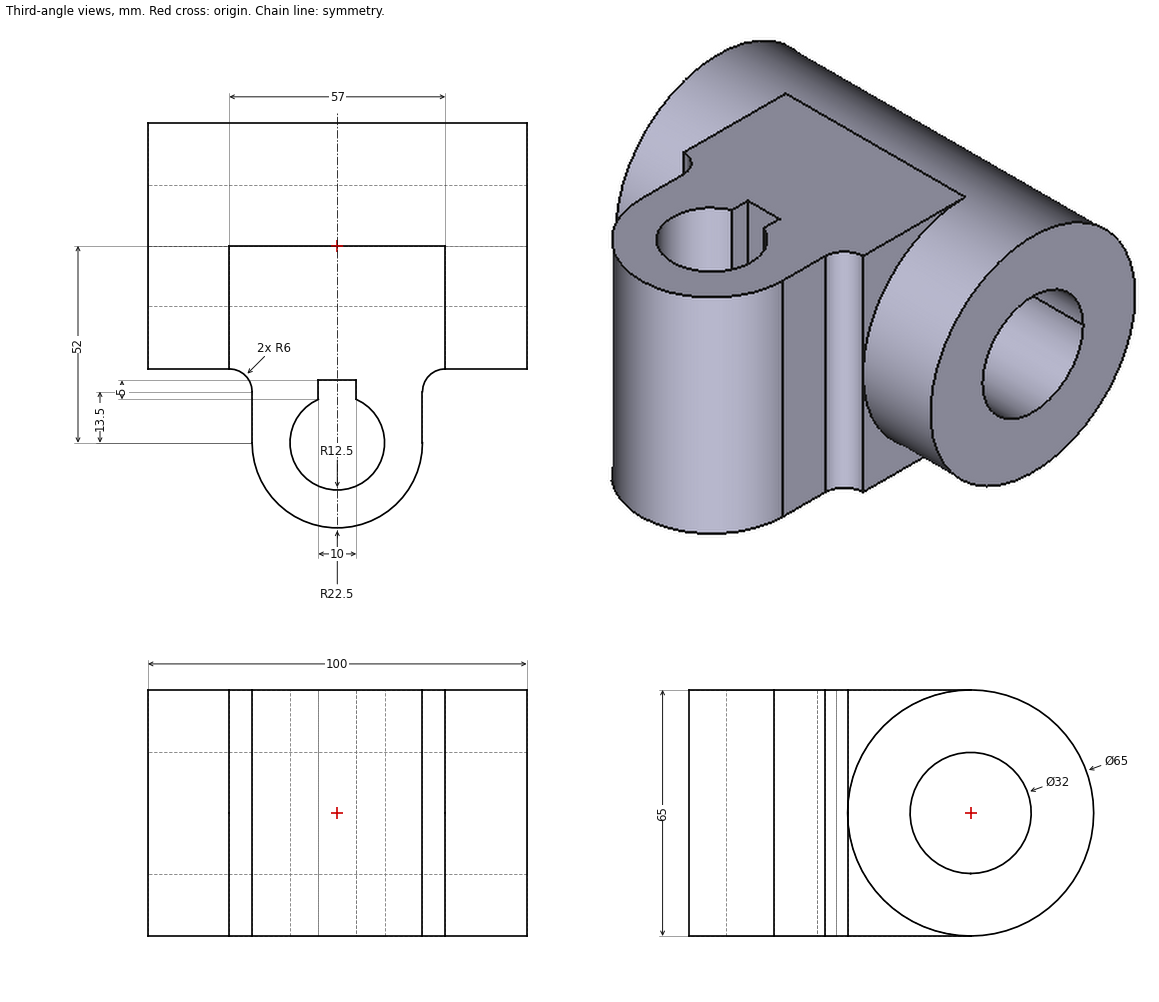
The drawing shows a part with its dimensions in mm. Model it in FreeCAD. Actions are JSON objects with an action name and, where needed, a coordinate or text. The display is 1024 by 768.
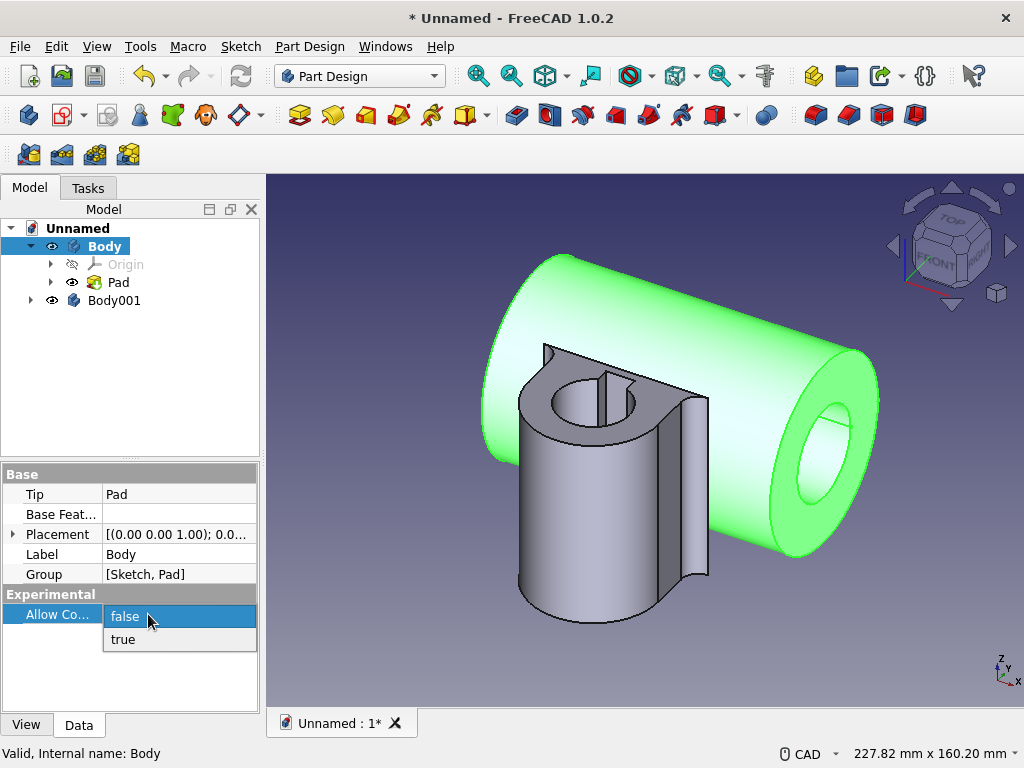
{"action": "left_click", "coordinate": [178, 640]}
{"action": "key", "text": "Return"}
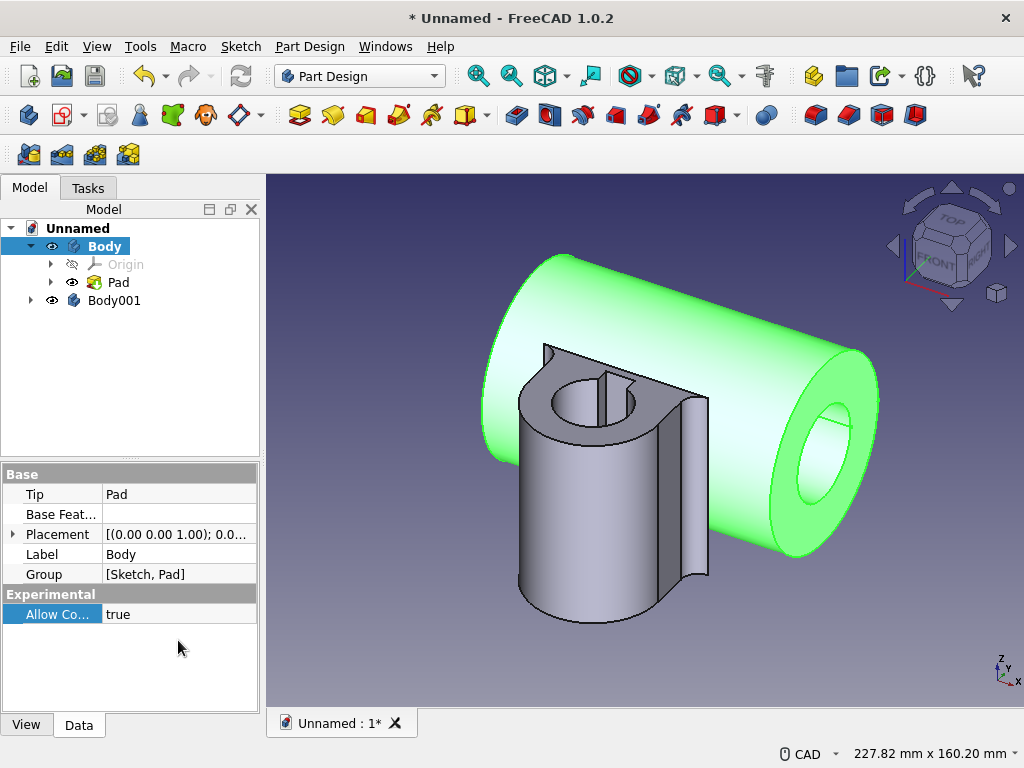
{"action": "left_click", "coordinate": [97, 300]}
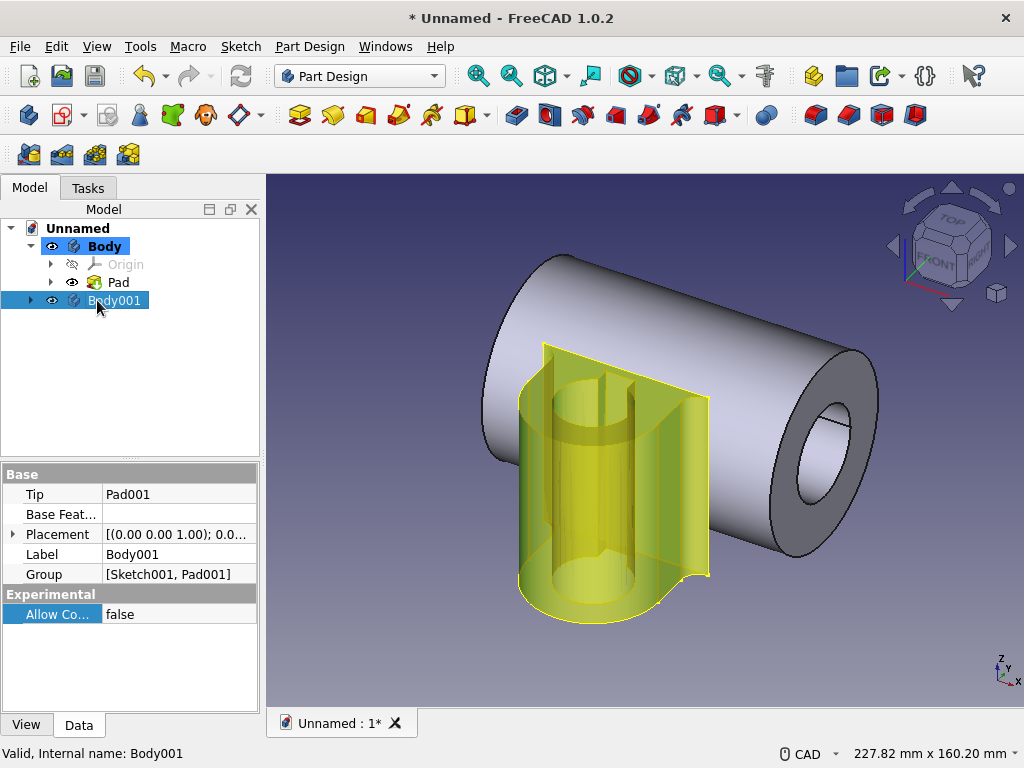
{"action": "left_click", "coordinate": [767, 116]}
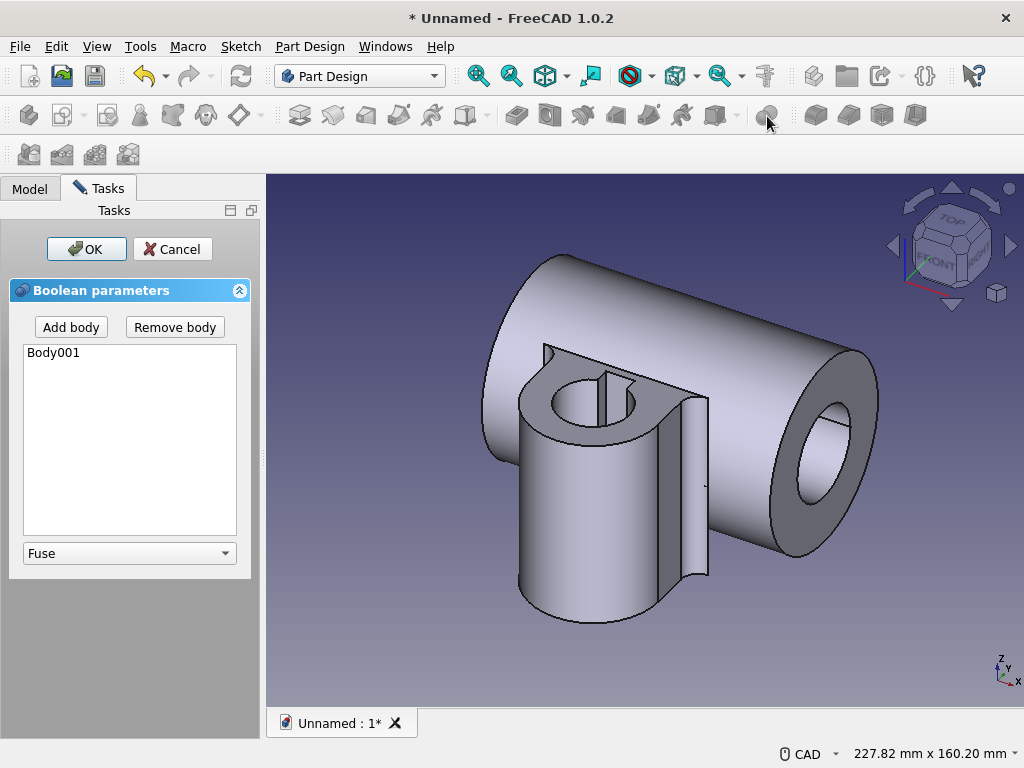
{"action": "left_click", "coordinate": [87, 249]}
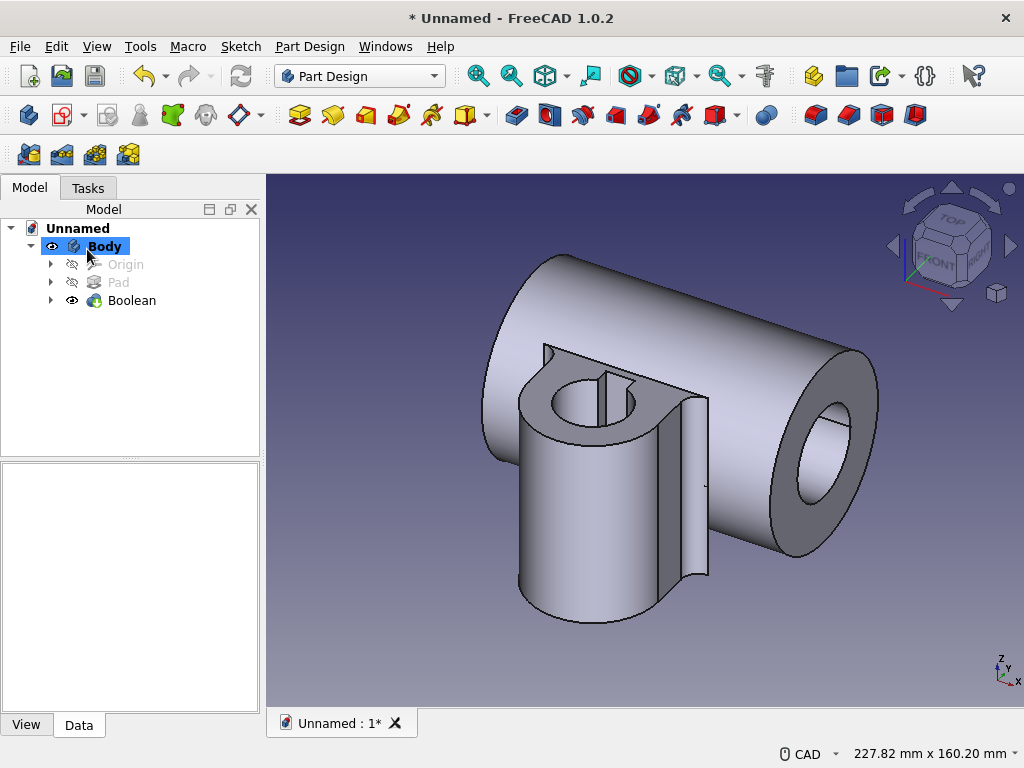
{"action": "left_click", "coordinate": [658, 400]}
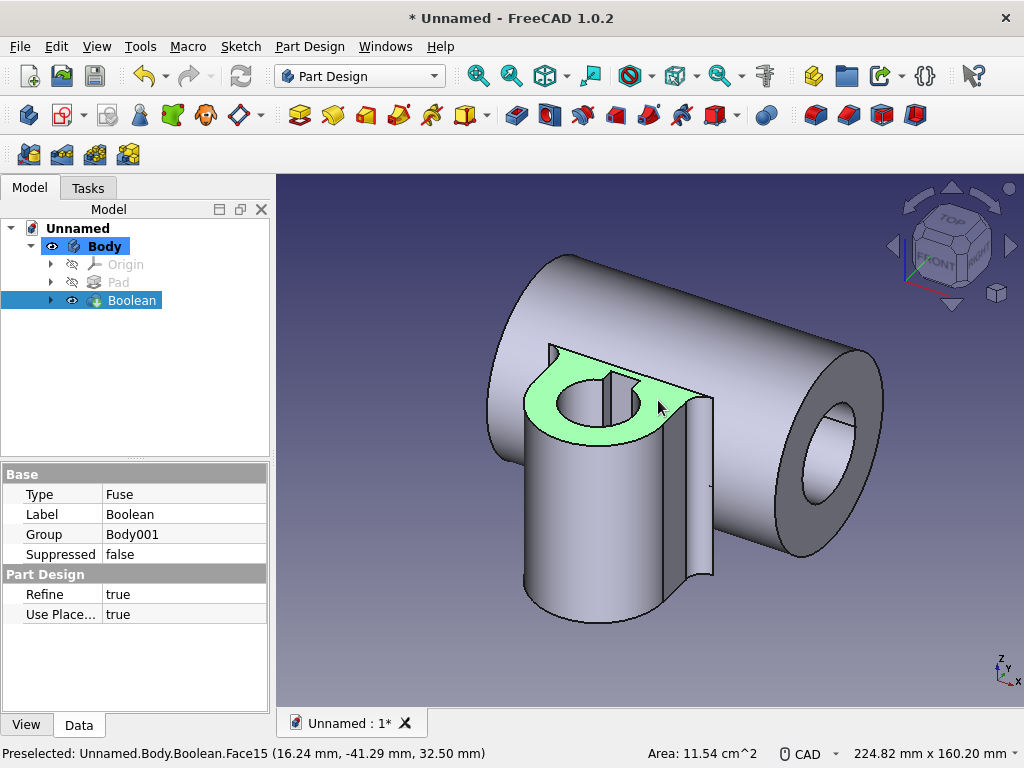
{"action": "left_click", "coordinate": [62, 116]}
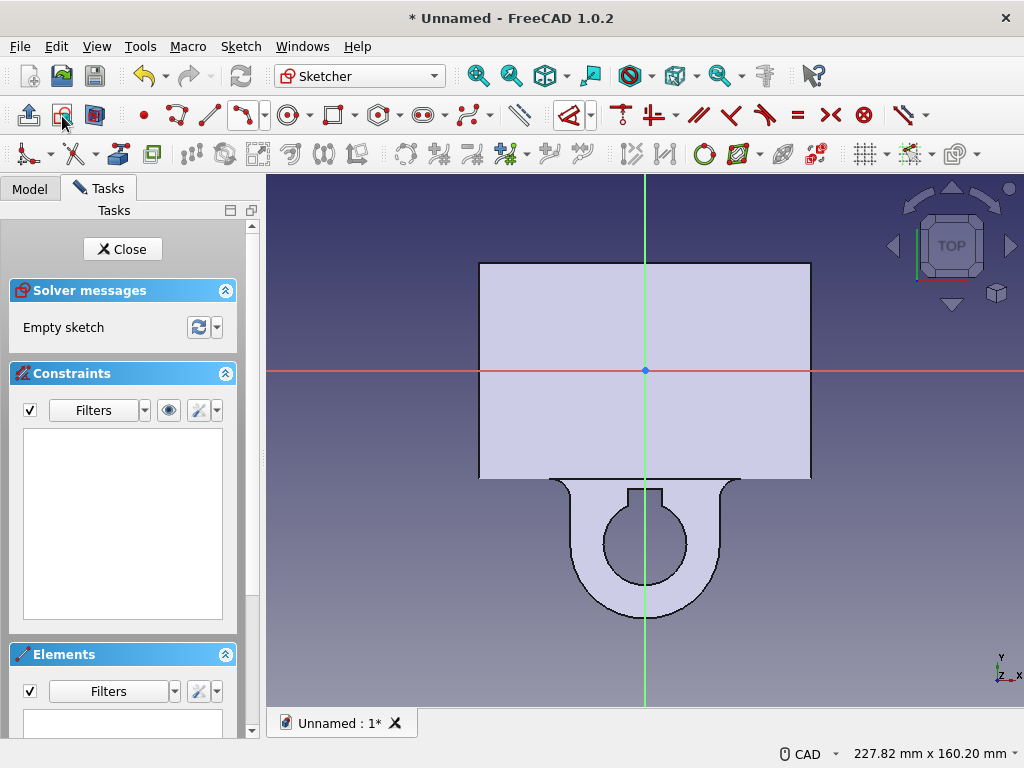
{"action": "scroll", "coordinate": [784, 605], "scroll_direction": "up", "scroll_amount": 2}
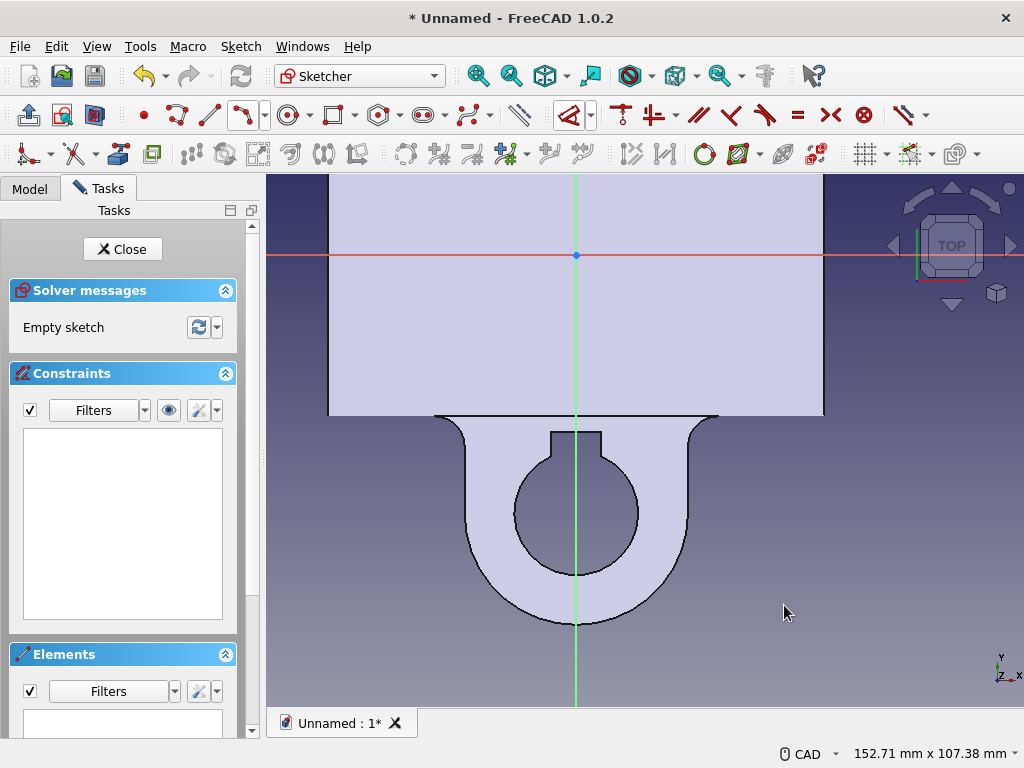
{"action": "key", "text": "g l"}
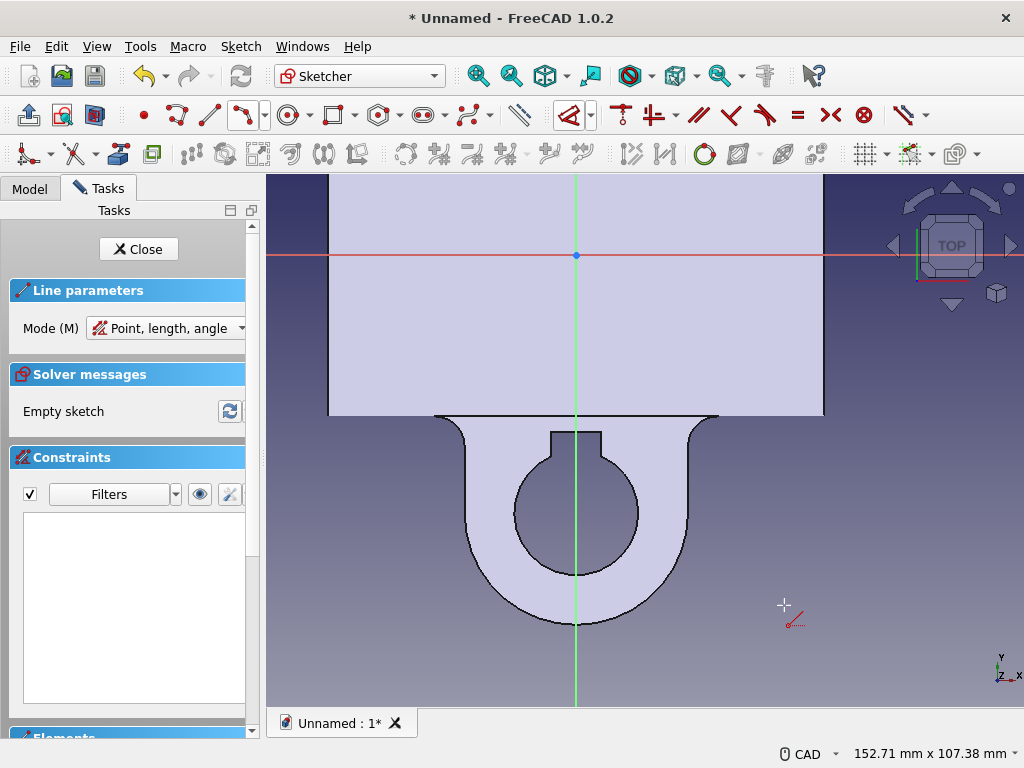
{"action": "left_click", "coordinate": [465, 446]}
{"action": "left_click", "coordinate": [465, 513]}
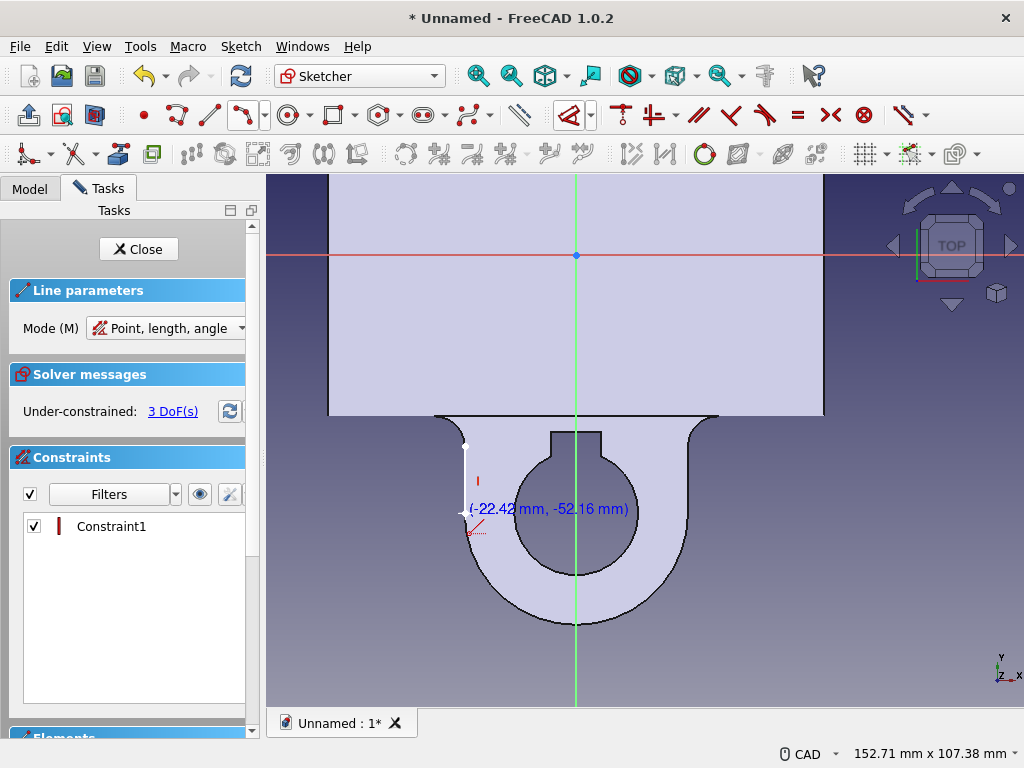
{"action": "left_click", "coordinate": [688, 513]}
{"action": "left_click", "coordinate": [688, 446]}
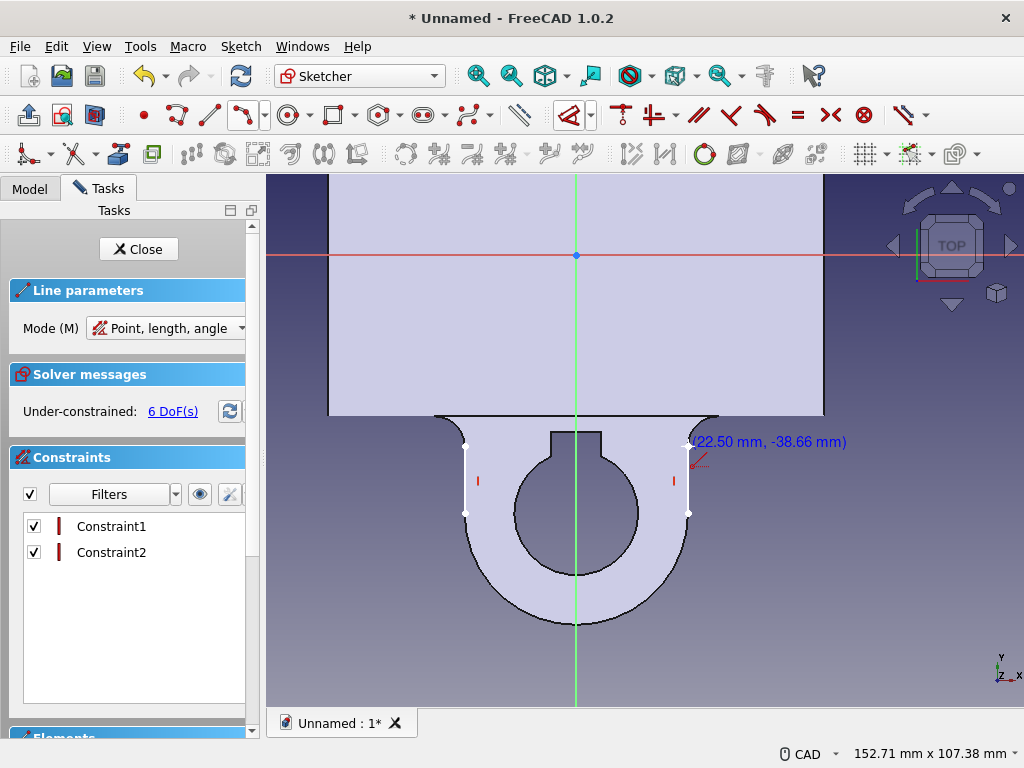
{"action": "left_click", "coordinate": [177, 116]}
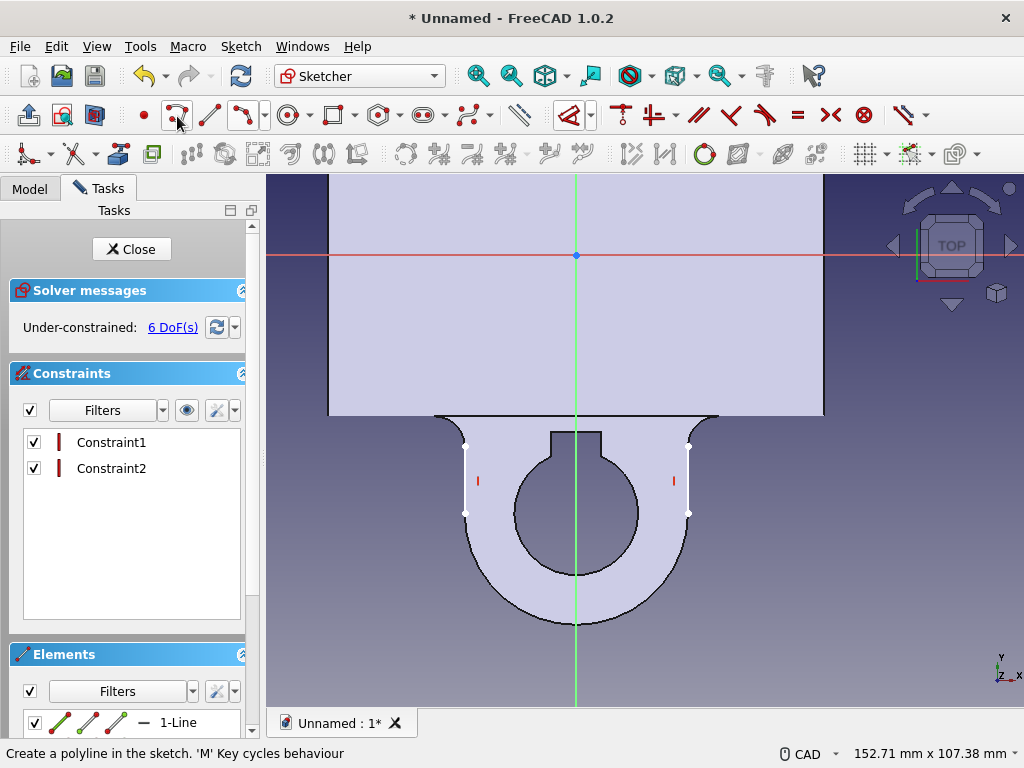
{"action": "left_click", "coordinate": [718, 416]}
{"action": "left_click", "coordinate": [718, 255]}
{"action": "left_click", "coordinate": [435, 264]}
{"action": "left_click", "coordinate": [435, 416]}
{"action": "right_click", "coordinate": [435, 416]}